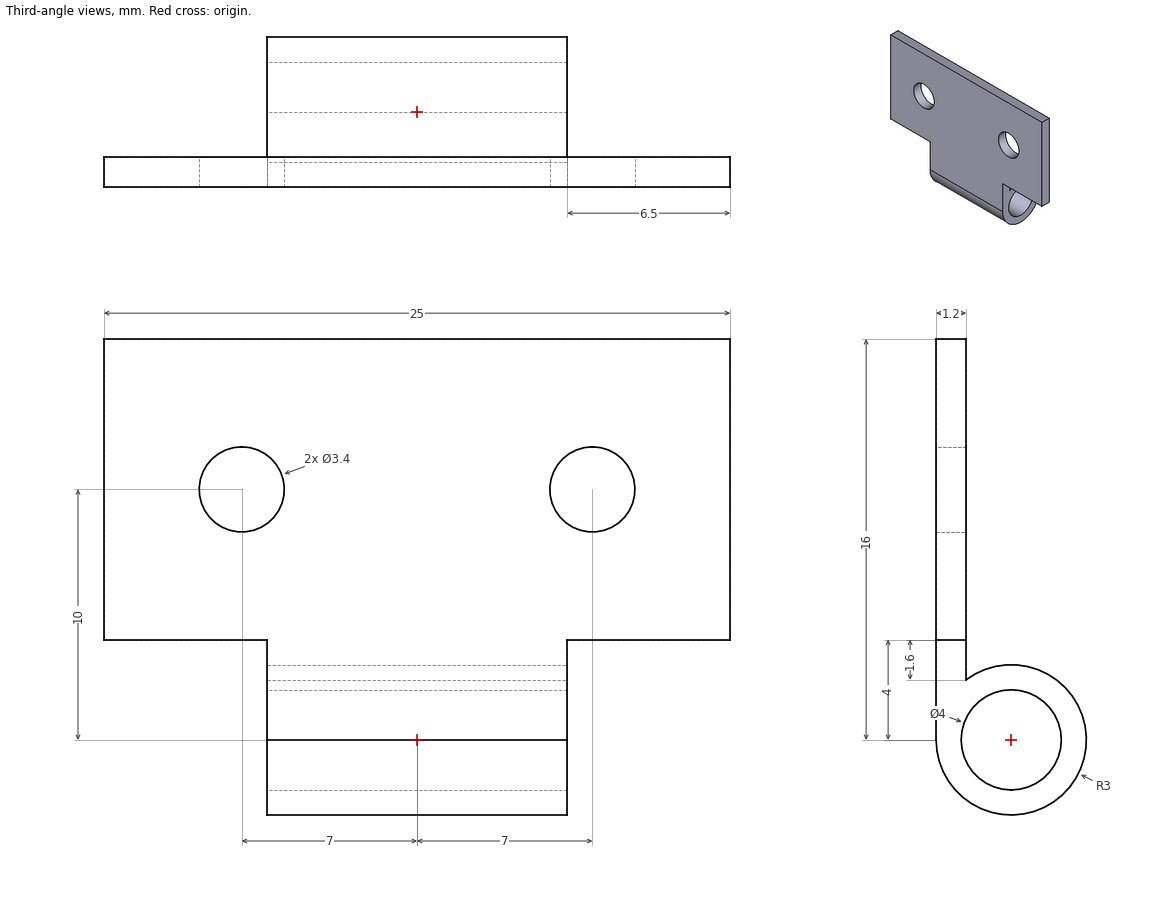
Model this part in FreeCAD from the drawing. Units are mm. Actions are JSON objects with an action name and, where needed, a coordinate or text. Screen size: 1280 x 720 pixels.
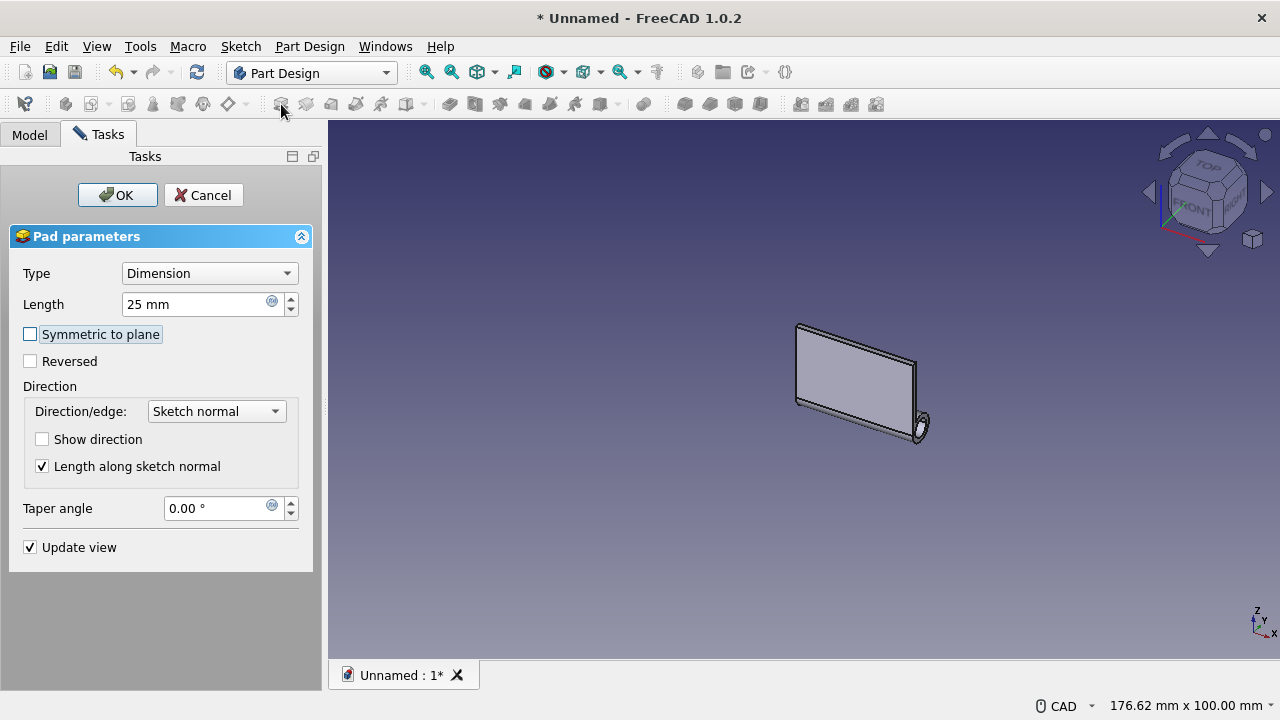
{"action": "left_click", "coordinate": [31, 334]}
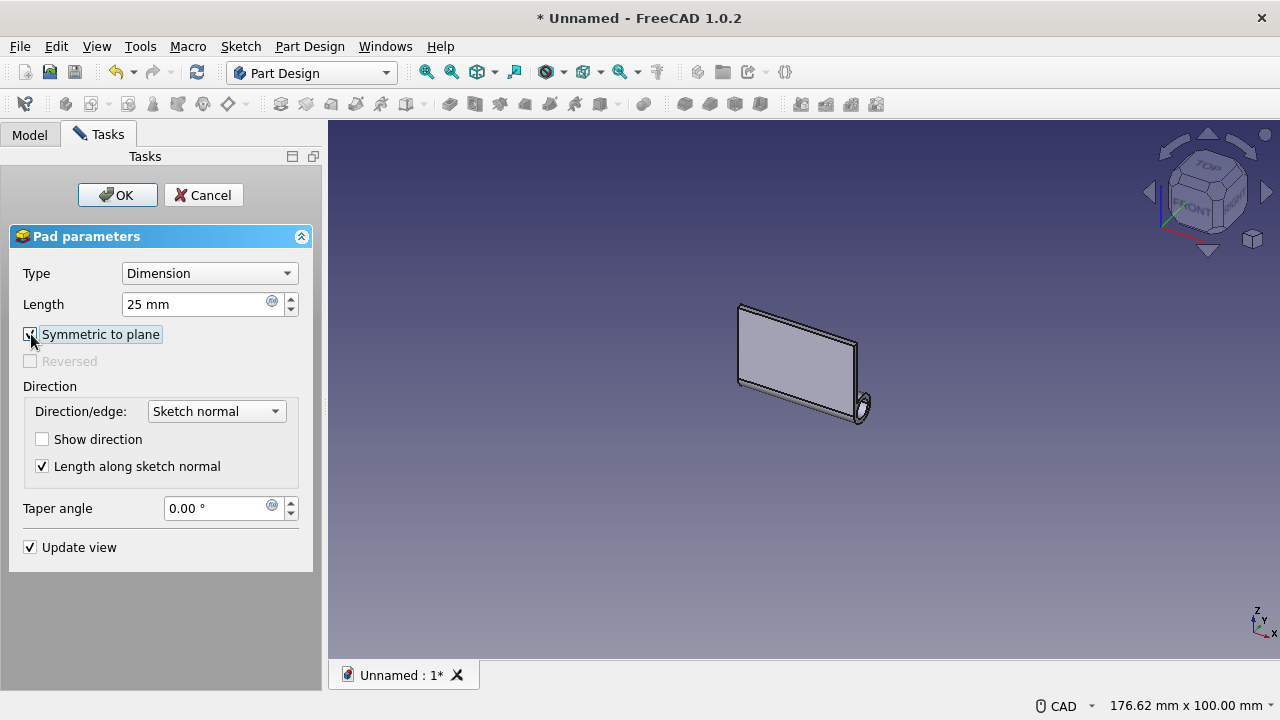
{"action": "left_click", "coordinate": [118, 195]}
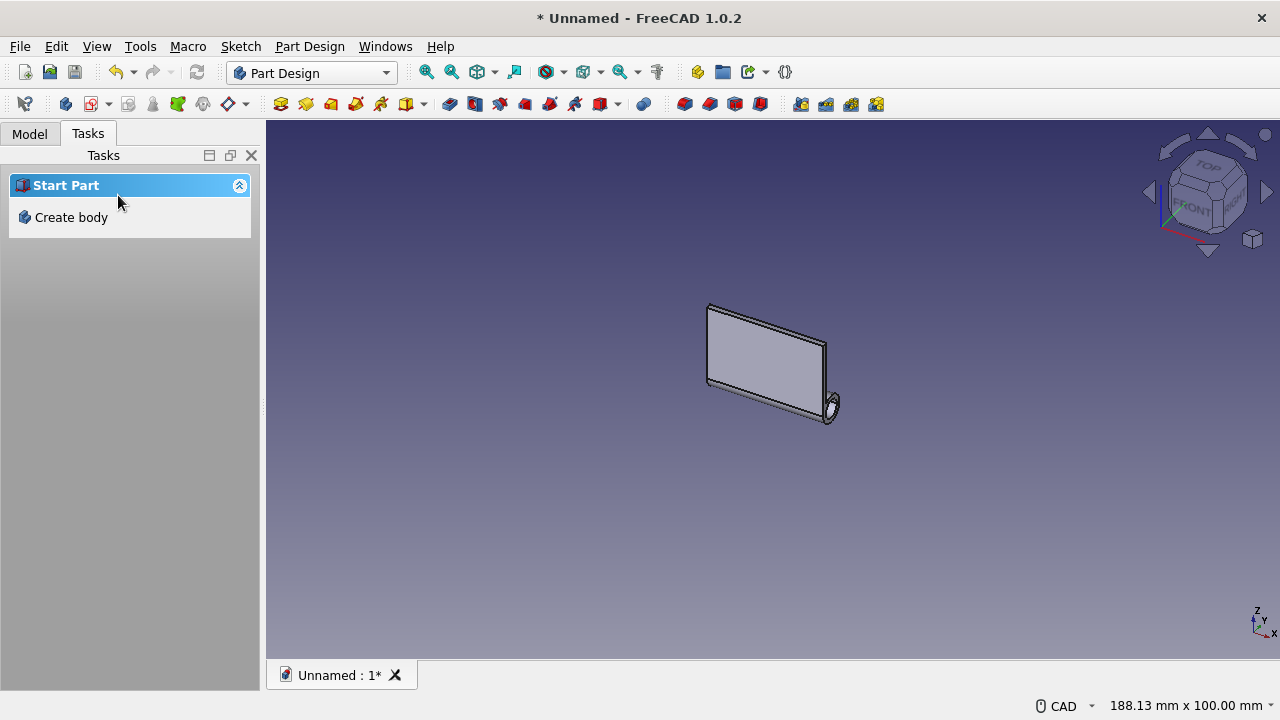
{"action": "left_click", "coordinate": [427, 72]}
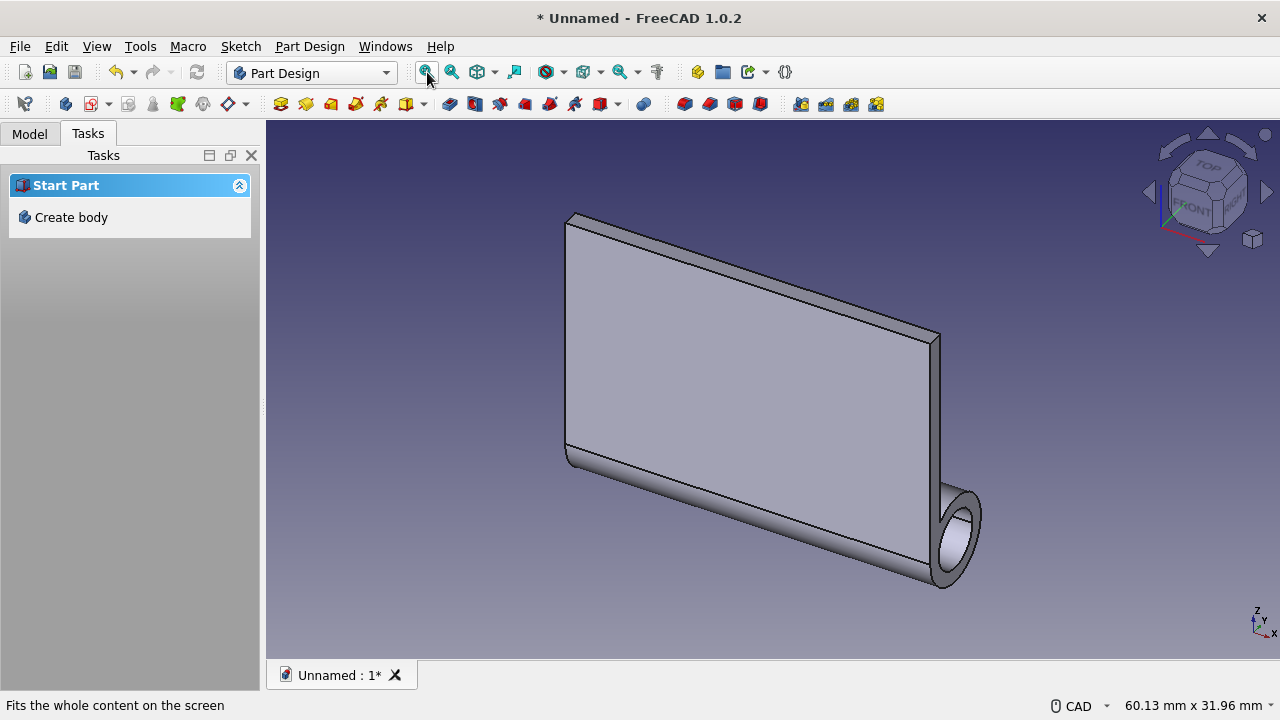
{"action": "key", "text": "4"}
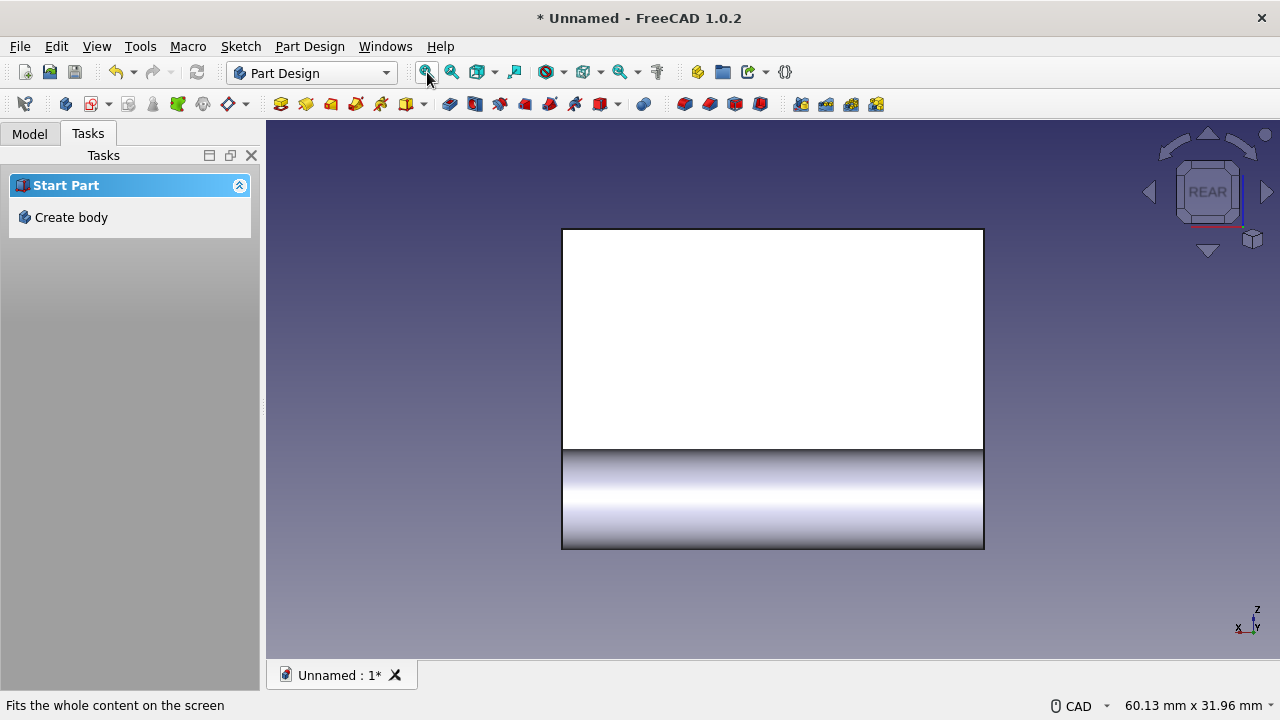
{"action": "left_click", "coordinate": [713, 343]}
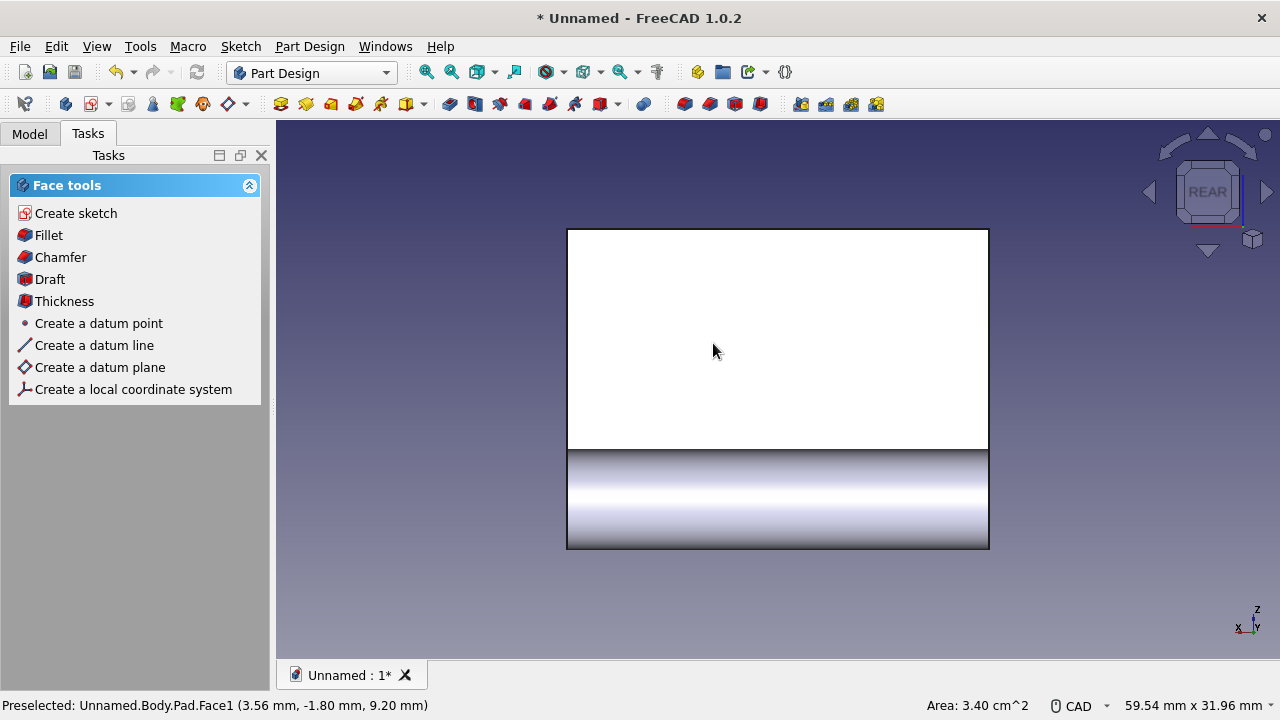
{"action": "left_click", "coordinate": [90, 104]}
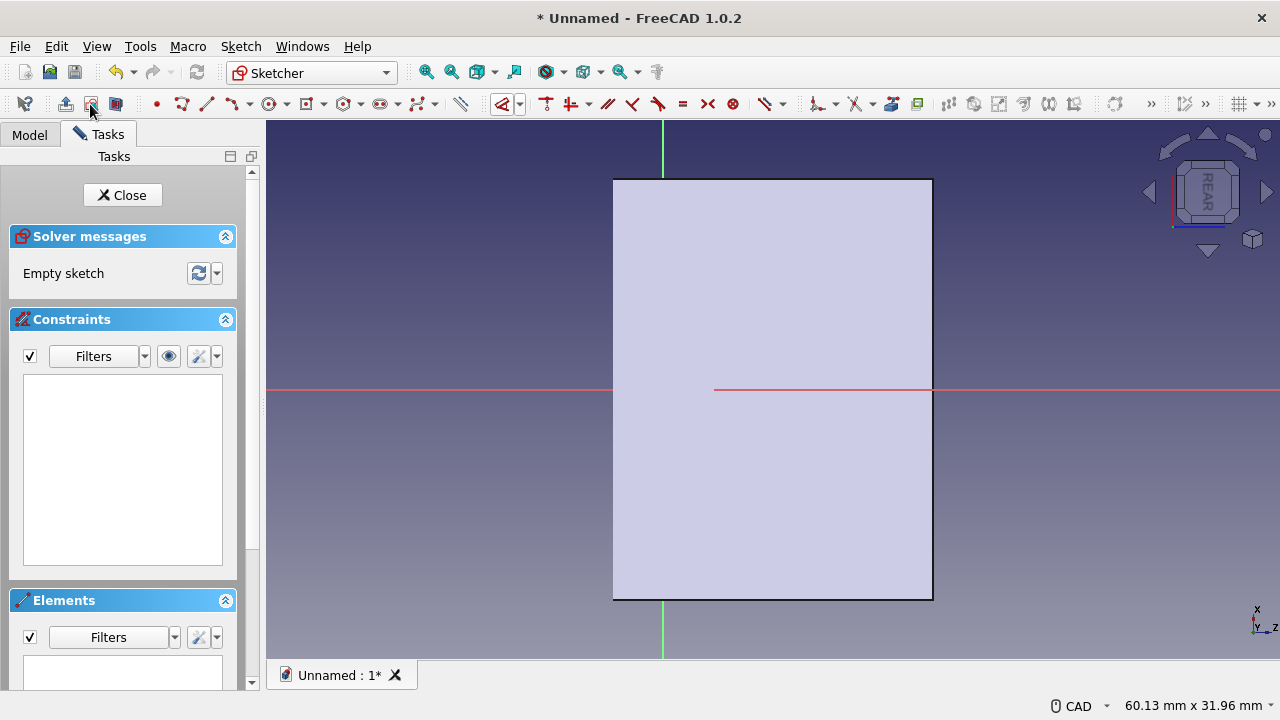
{"action": "left_click", "coordinate": [116, 104]}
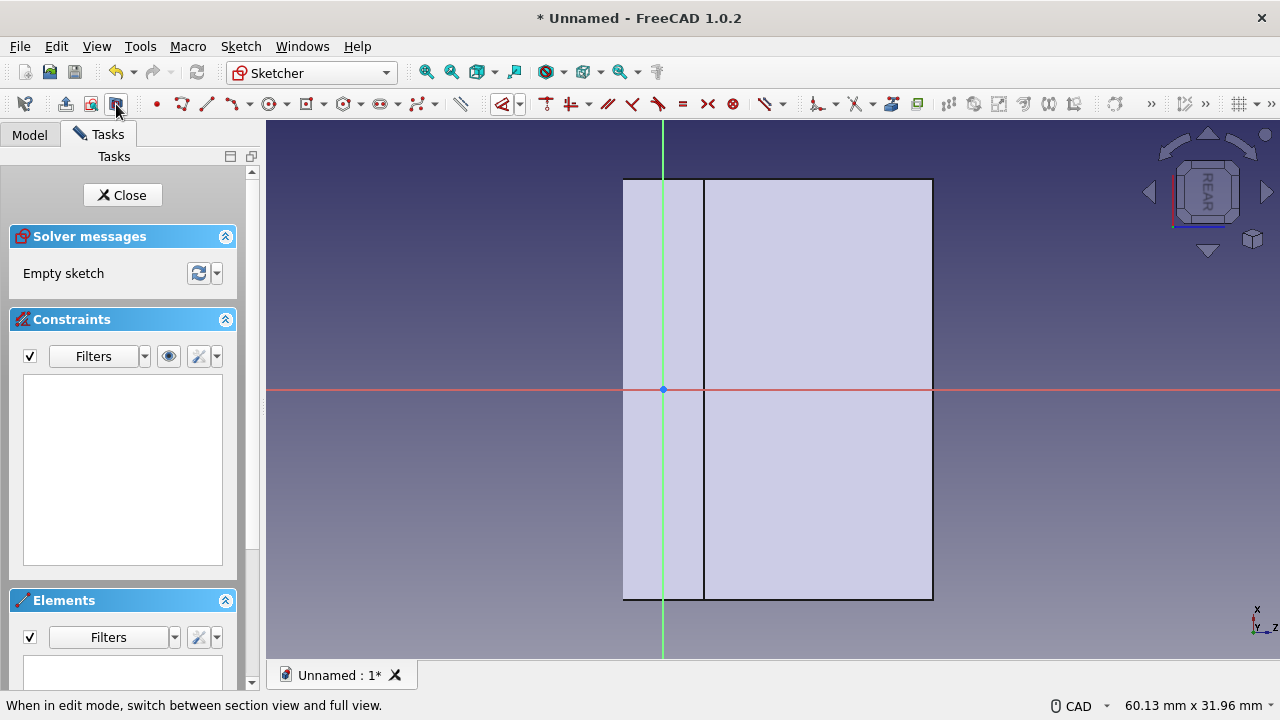
{"action": "left_click", "coordinate": [268, 104]}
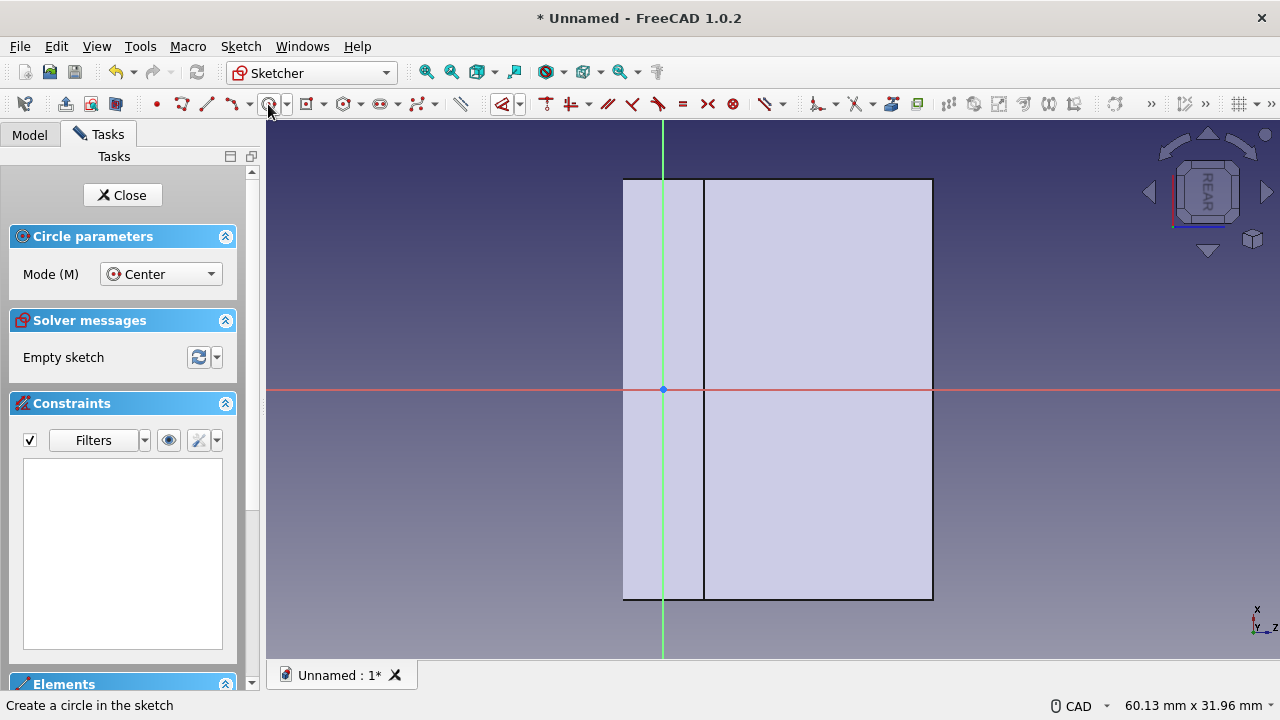
{"action": "left_click", "coordinate": [832, 508]}
{"action": "mouse_move", "coordinate": [852, 487]}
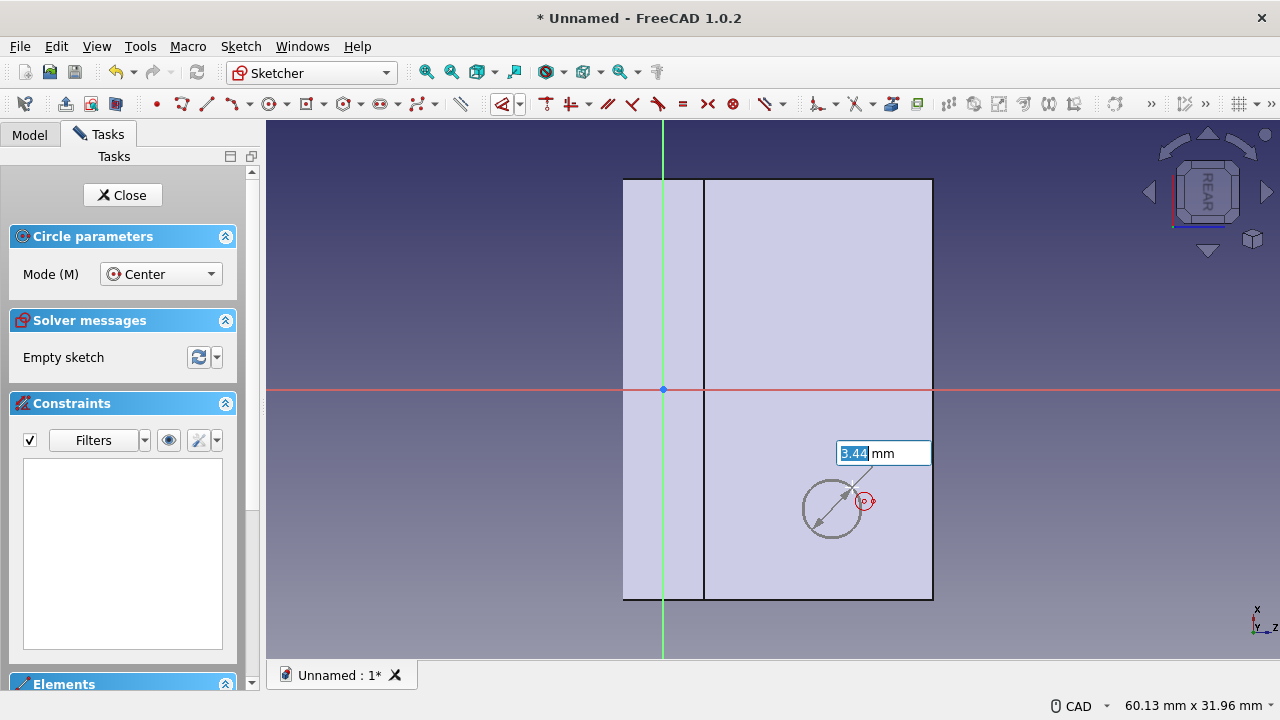
{"action": "type", "text": "3.4"}
{"action": "key", "text": "Return"}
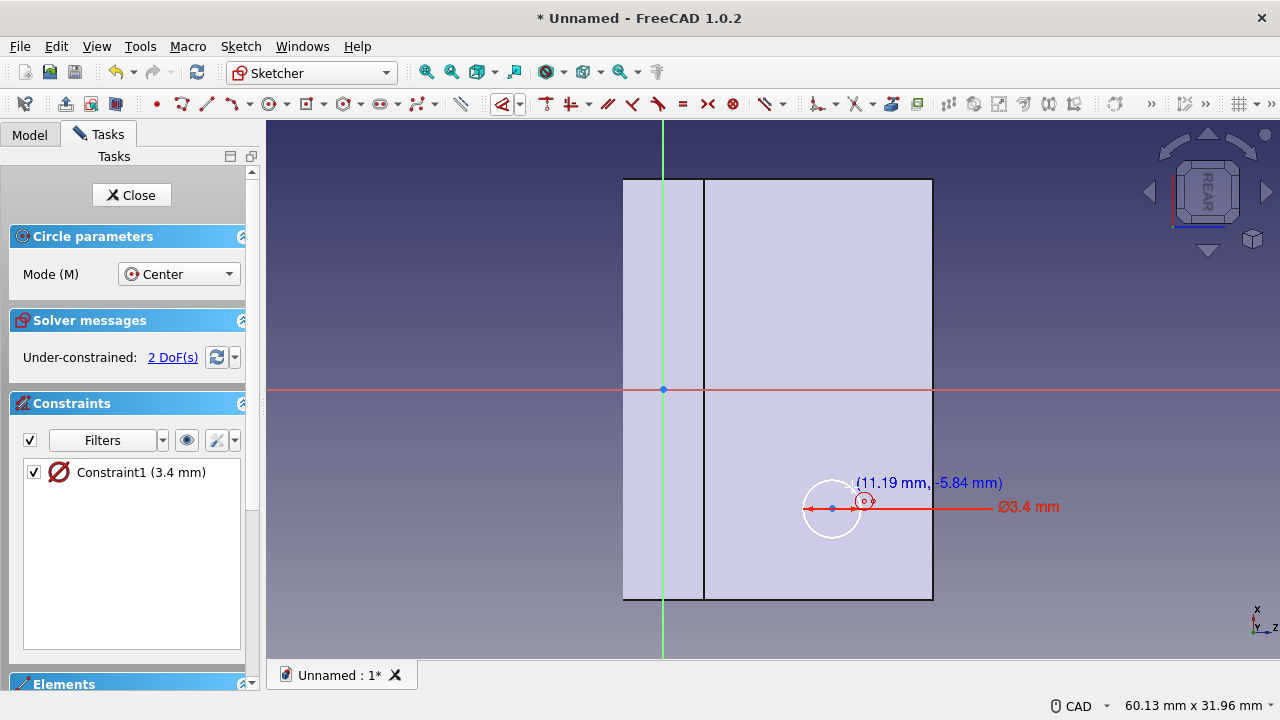
{"action": "left_click", "coordinate": [832, 271]}
{"action": "mouse_move", "coordinate": [852, 251]}